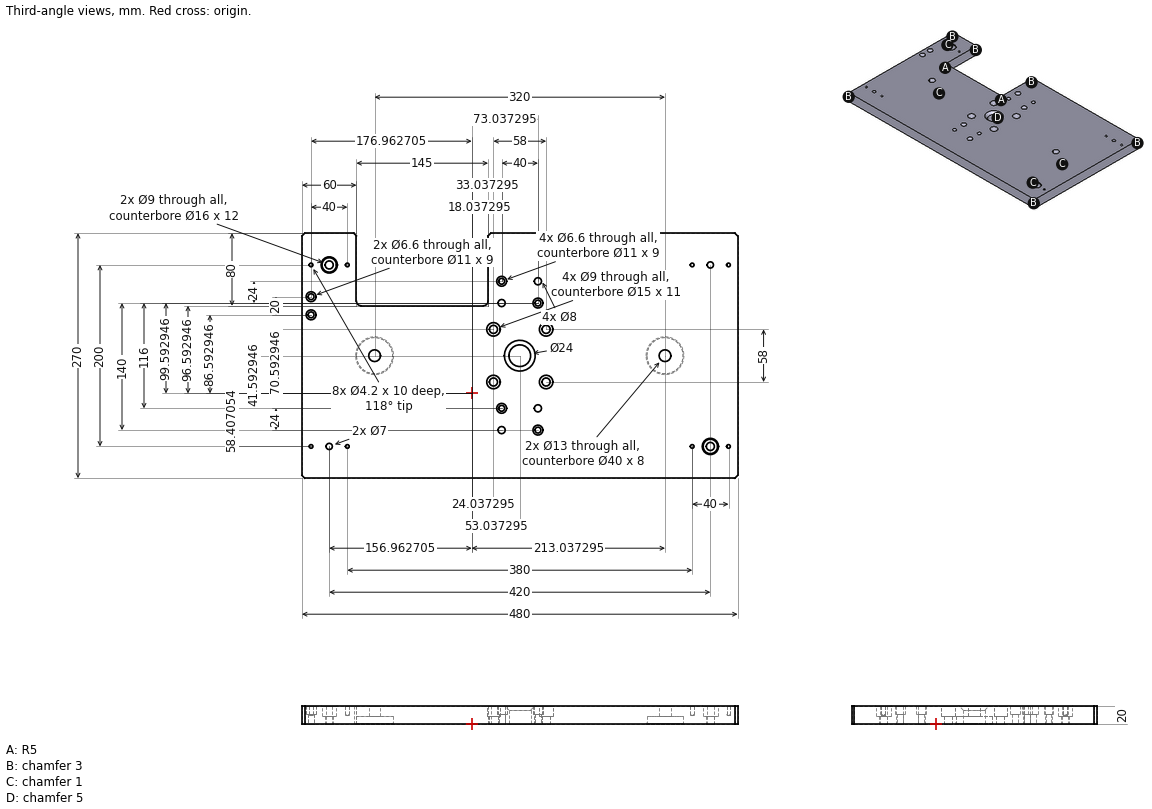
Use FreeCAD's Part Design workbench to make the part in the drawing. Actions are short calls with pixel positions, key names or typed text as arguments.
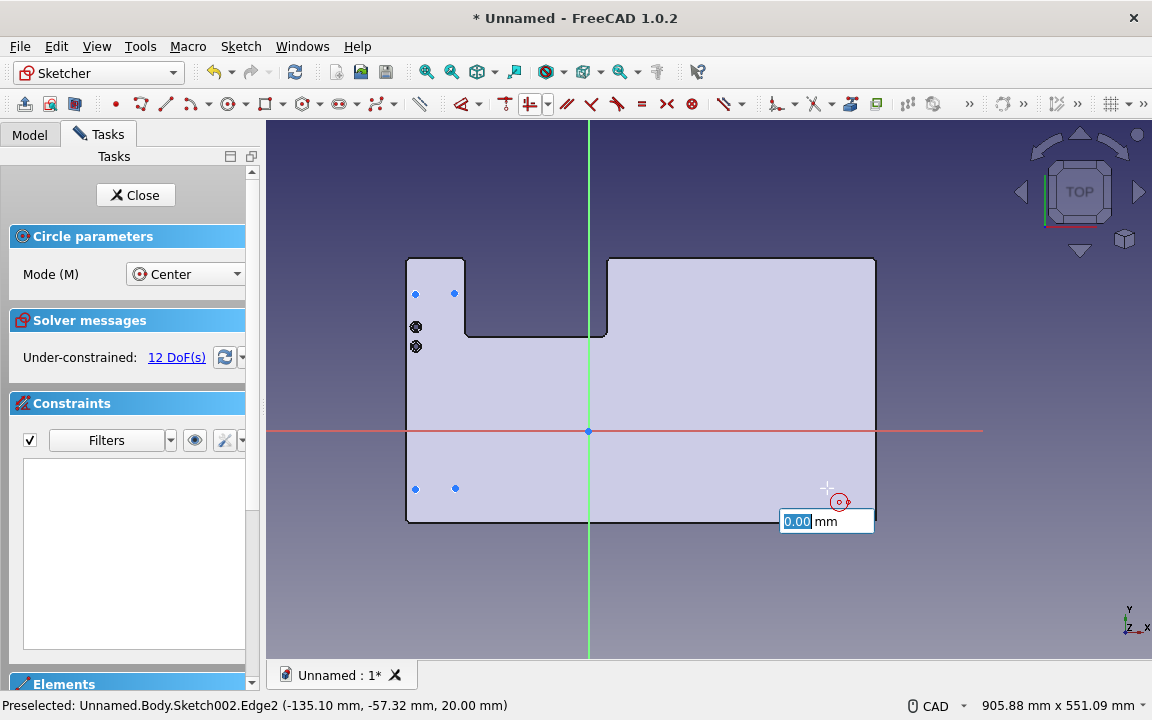
scroll(828, 487, up, 11)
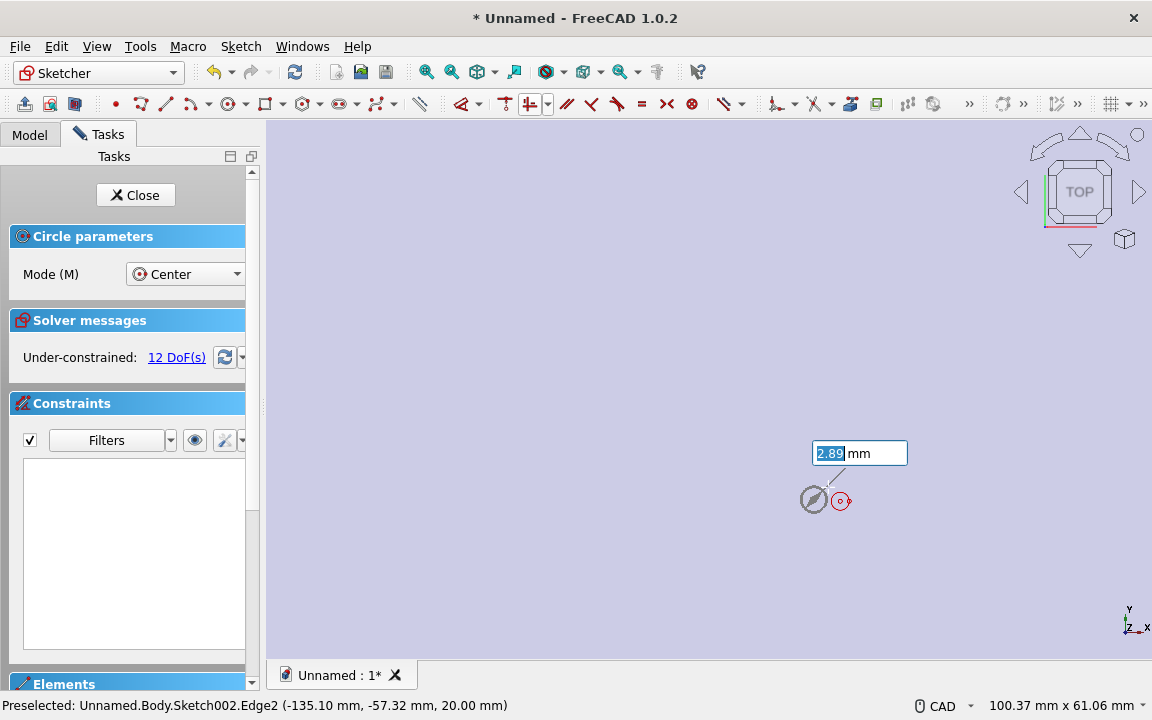
click(824, 480)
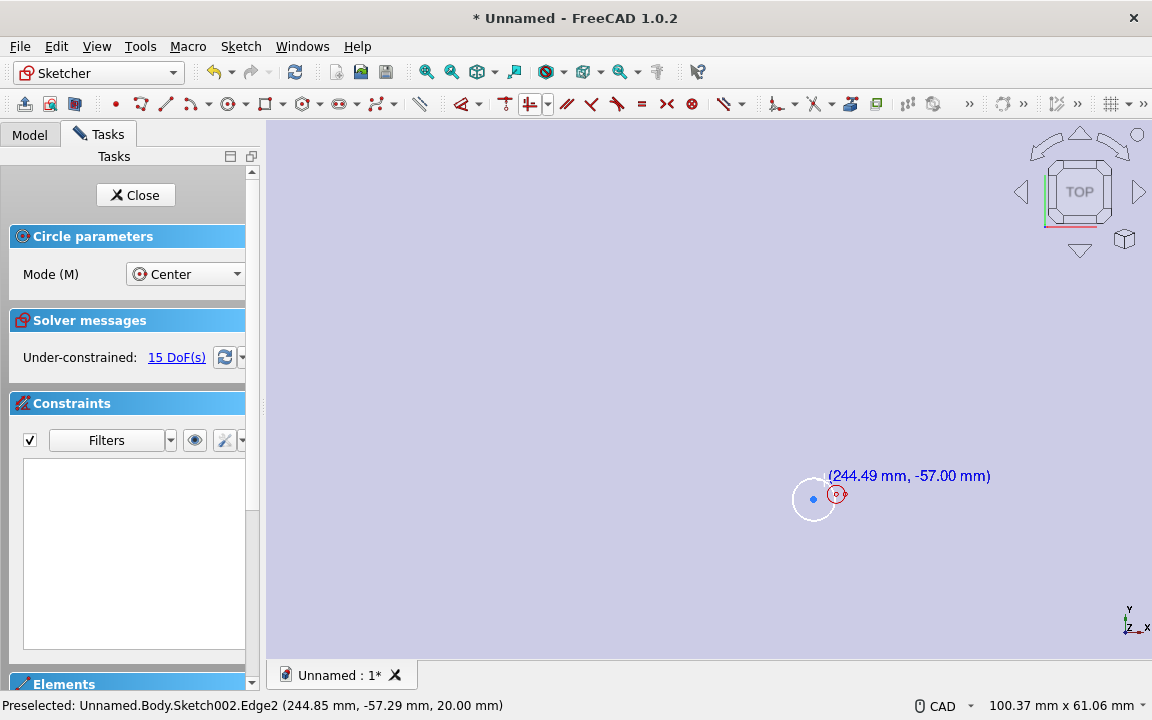
scroll(828, 487, down, 11)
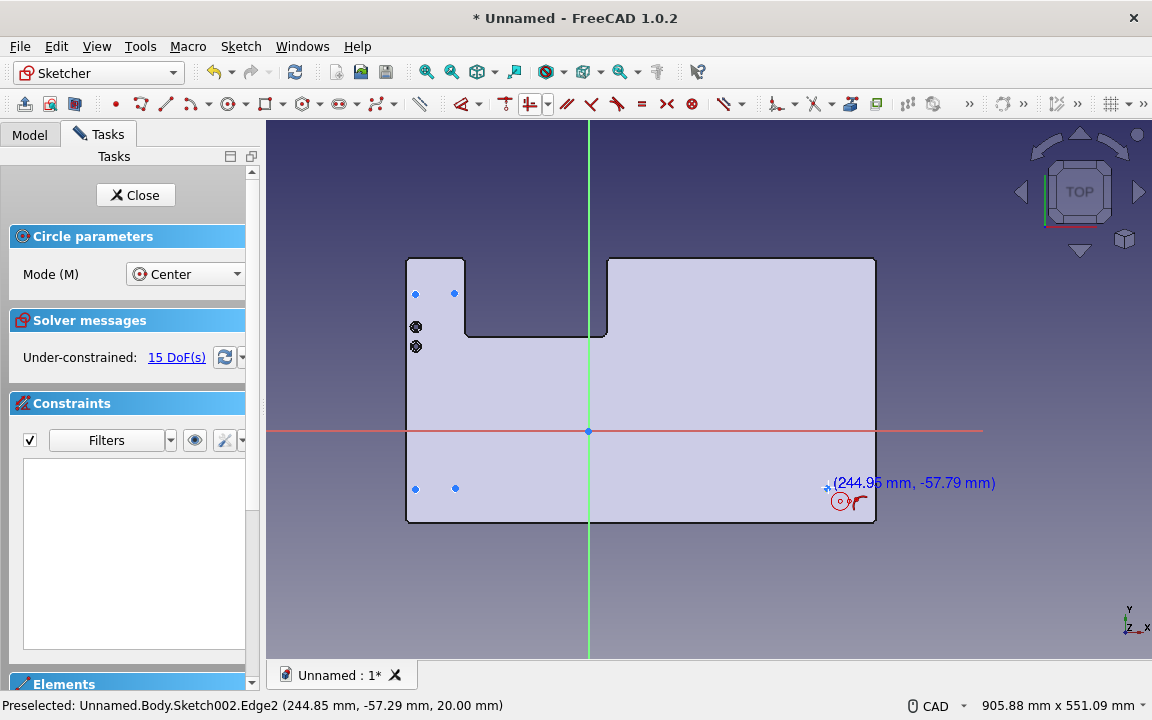
scroll(866, 488, up, 13)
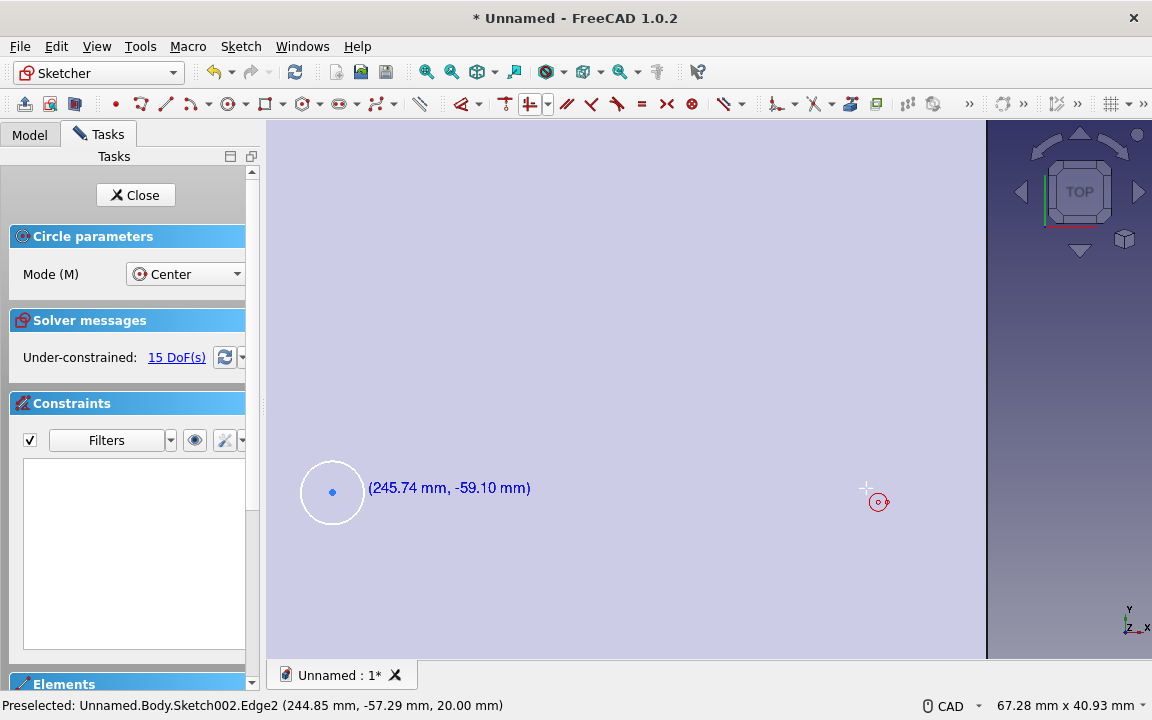
scroll(866, 488, down, 13)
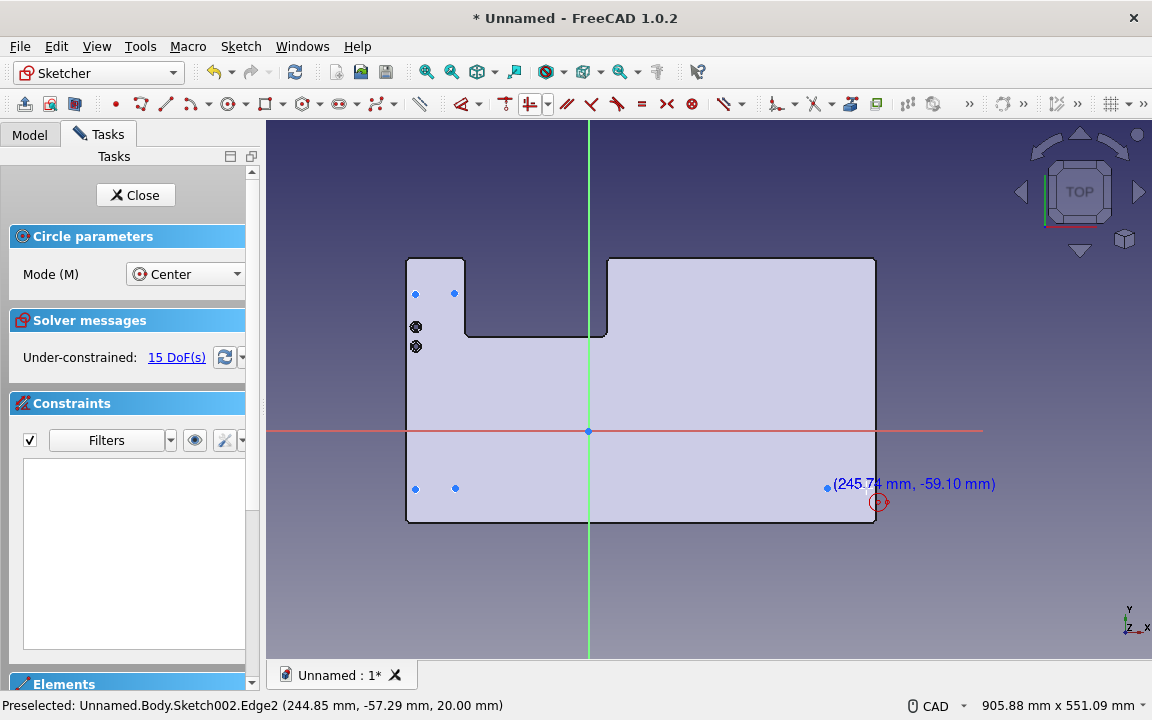
click(866, 488)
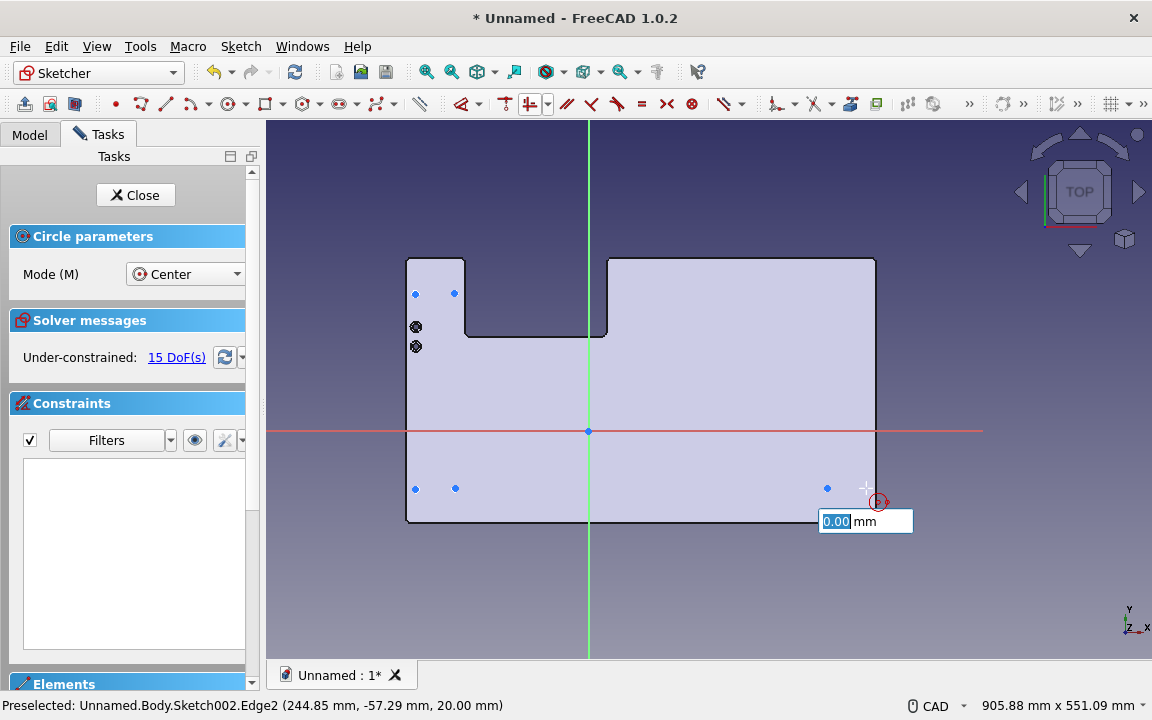
scroll(867, 487, up, 11)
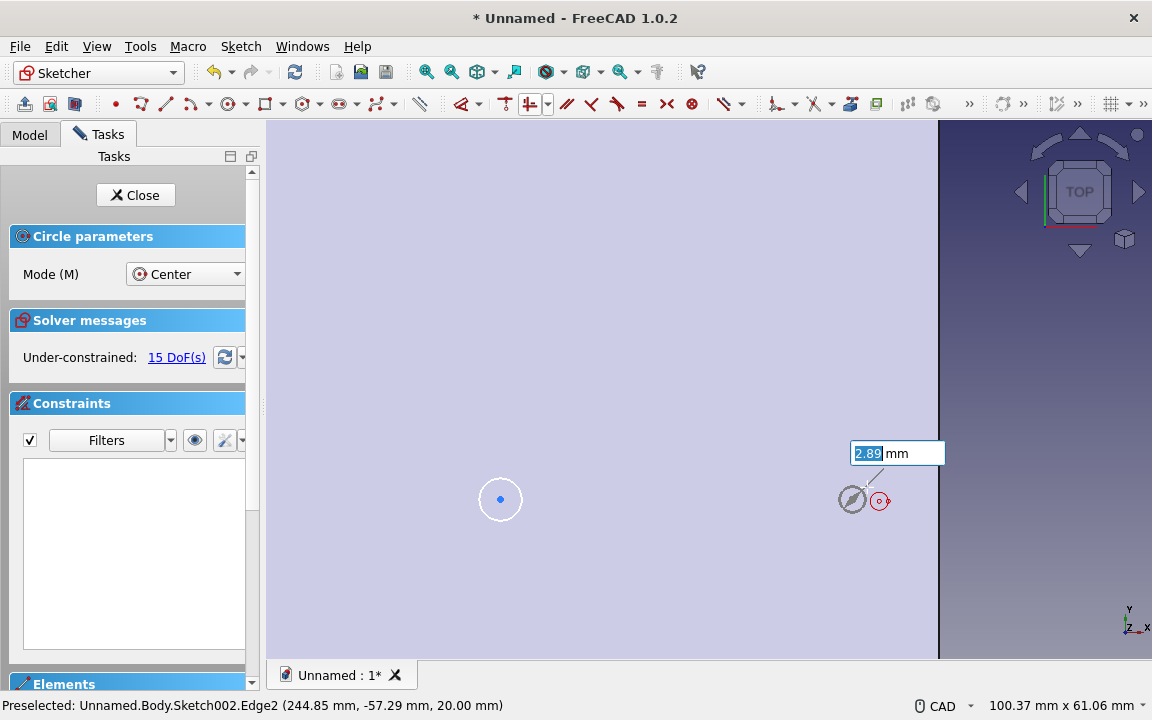
click(864, 480)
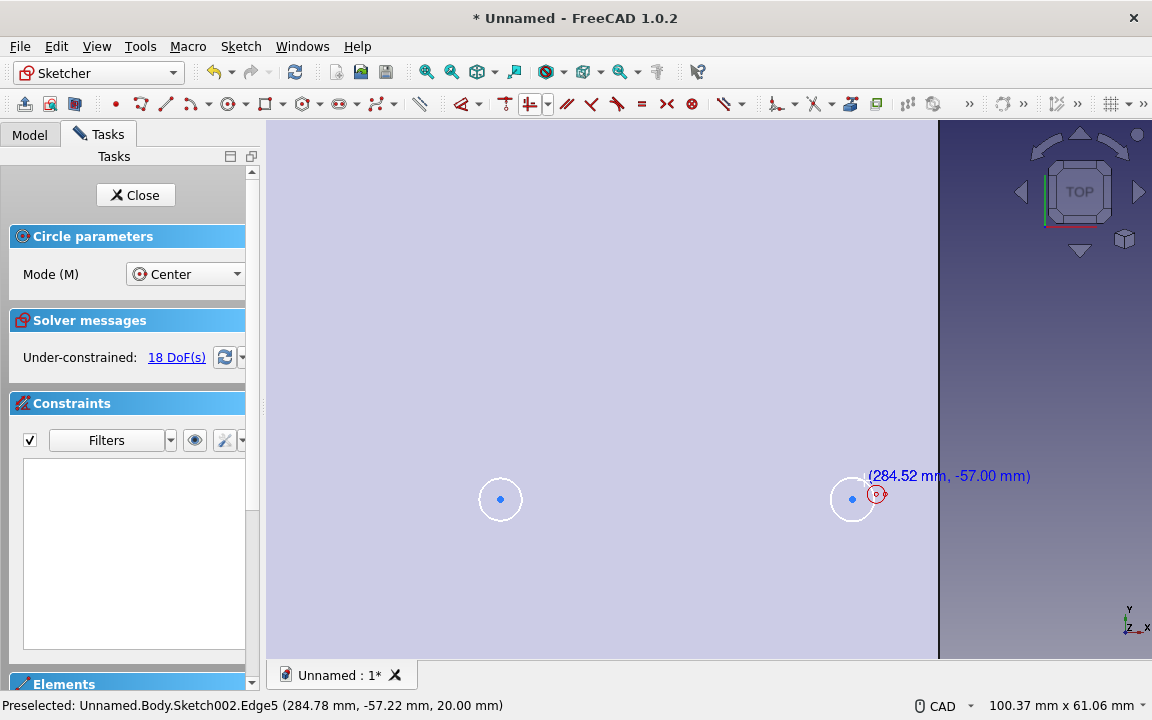
scroll(867, 487, down, 11)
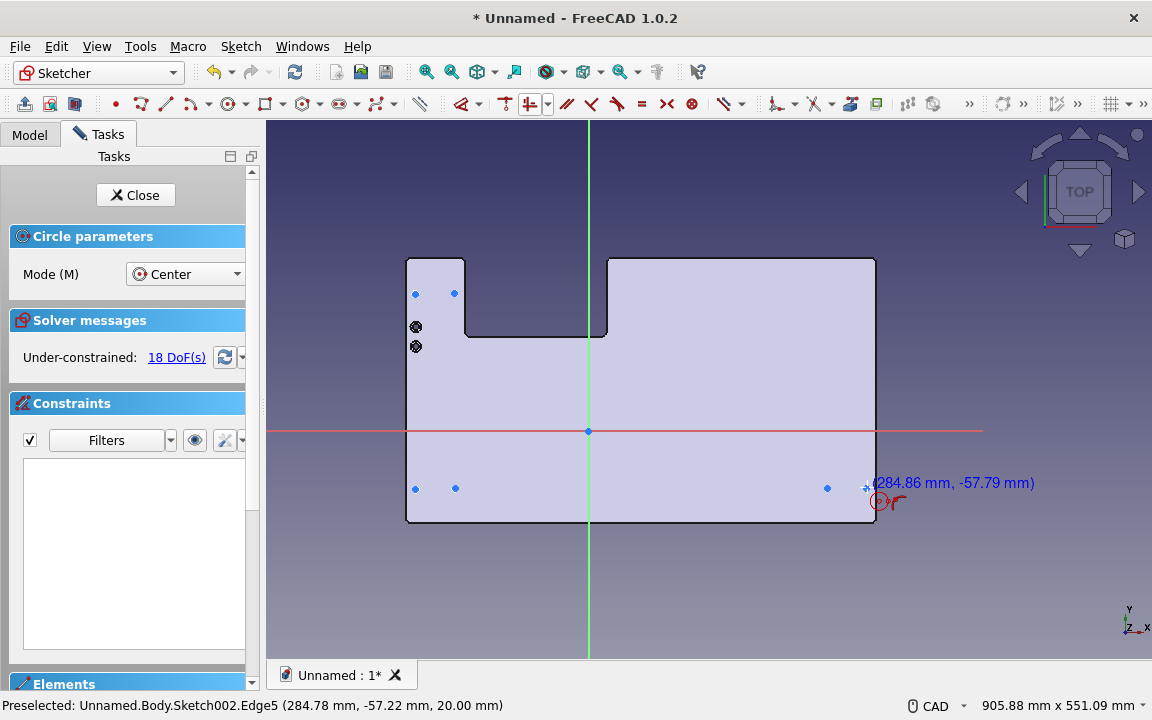
scroll(866, 293, up, 13)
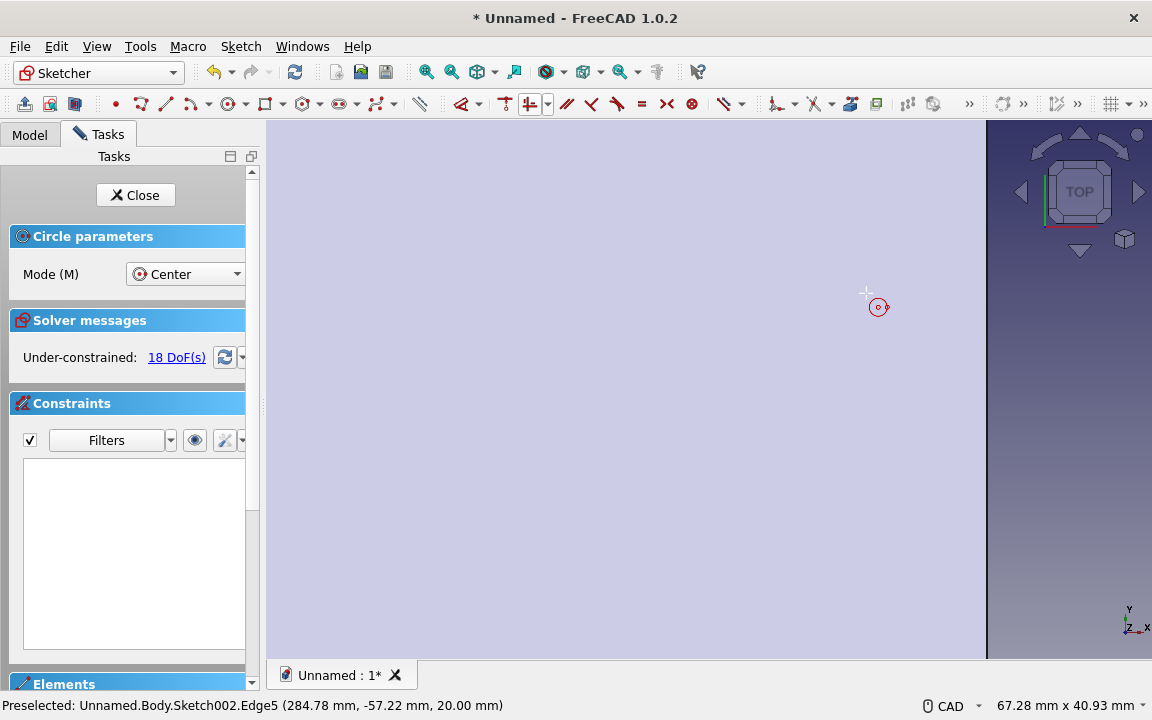
scroll(866, 292, down, 13)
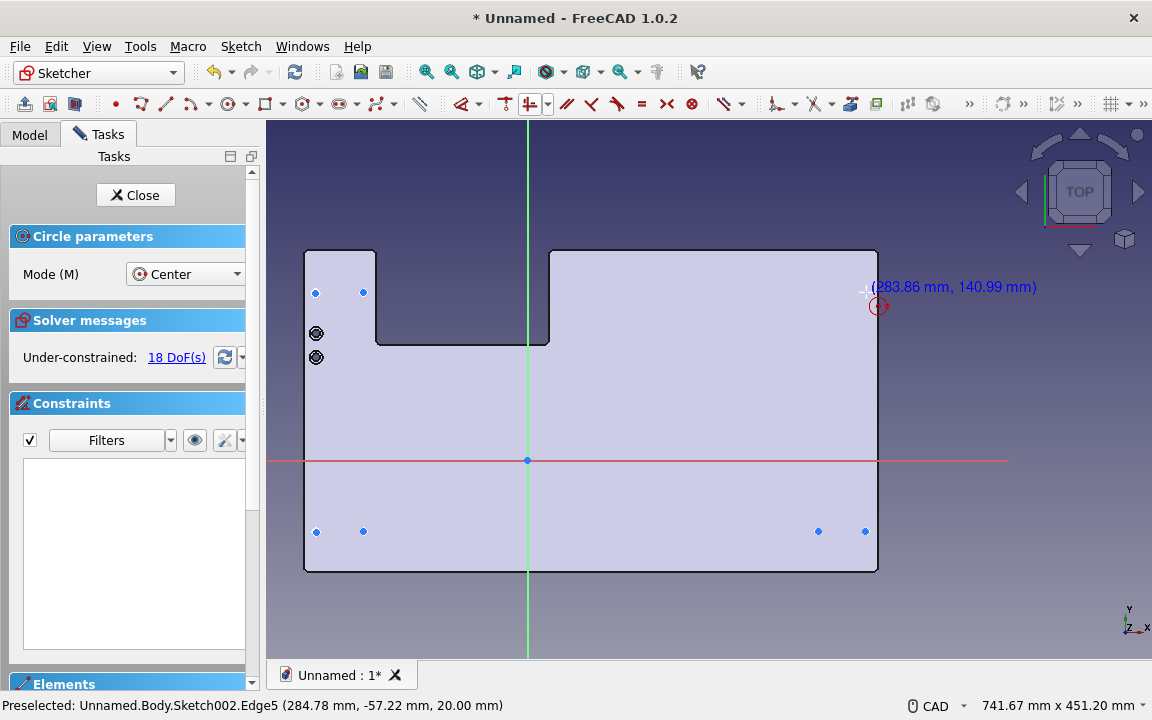
click(866, 292)